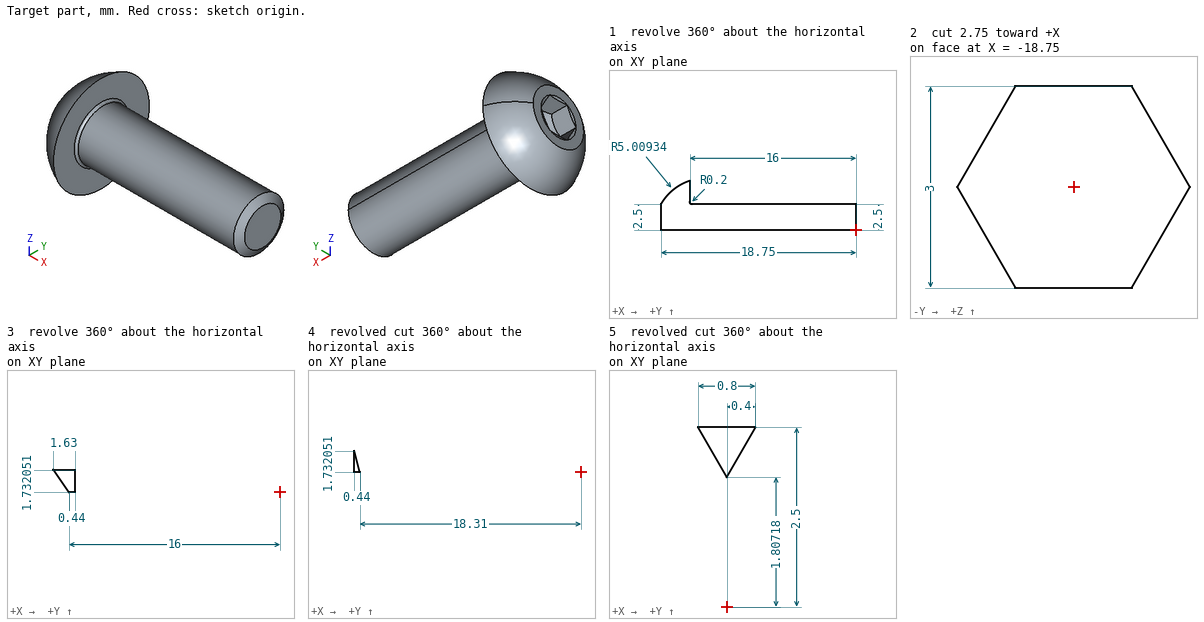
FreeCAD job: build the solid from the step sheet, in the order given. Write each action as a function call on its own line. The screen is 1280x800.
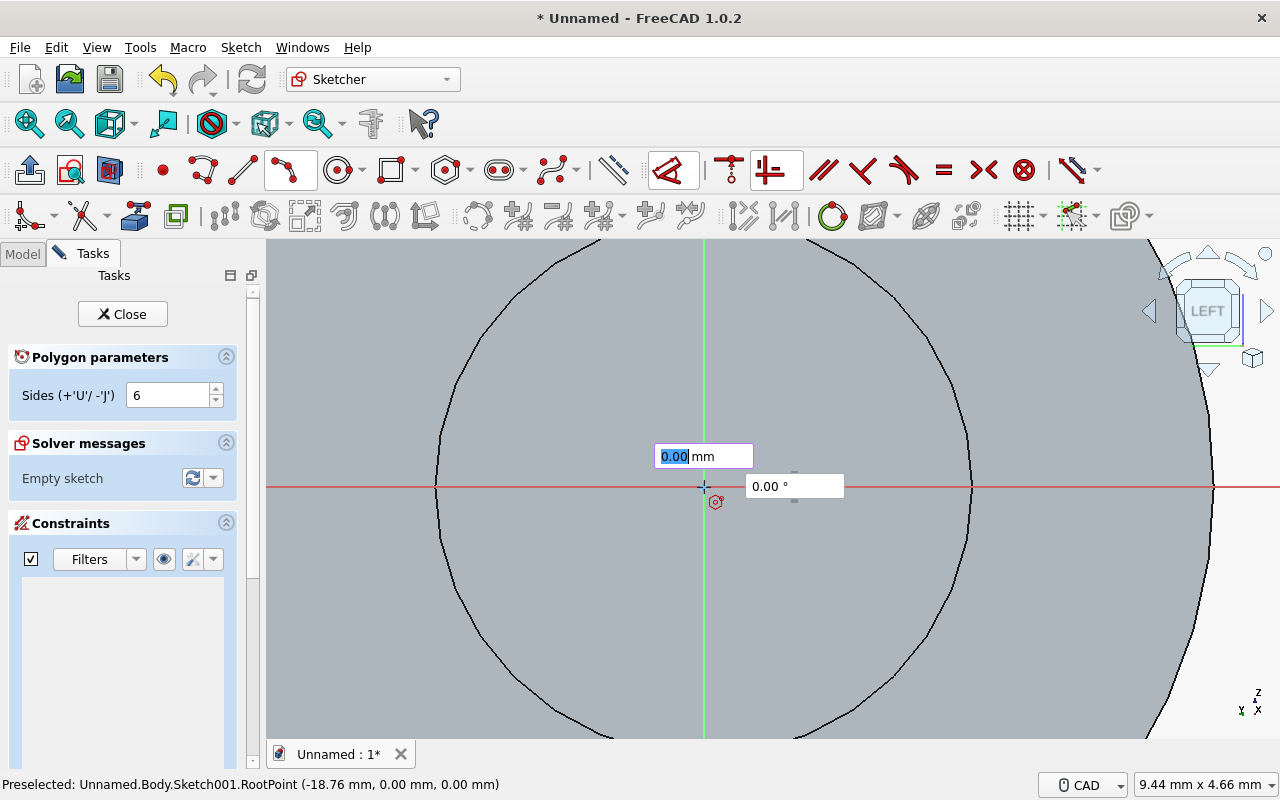
click(518, 487)
key(Escape)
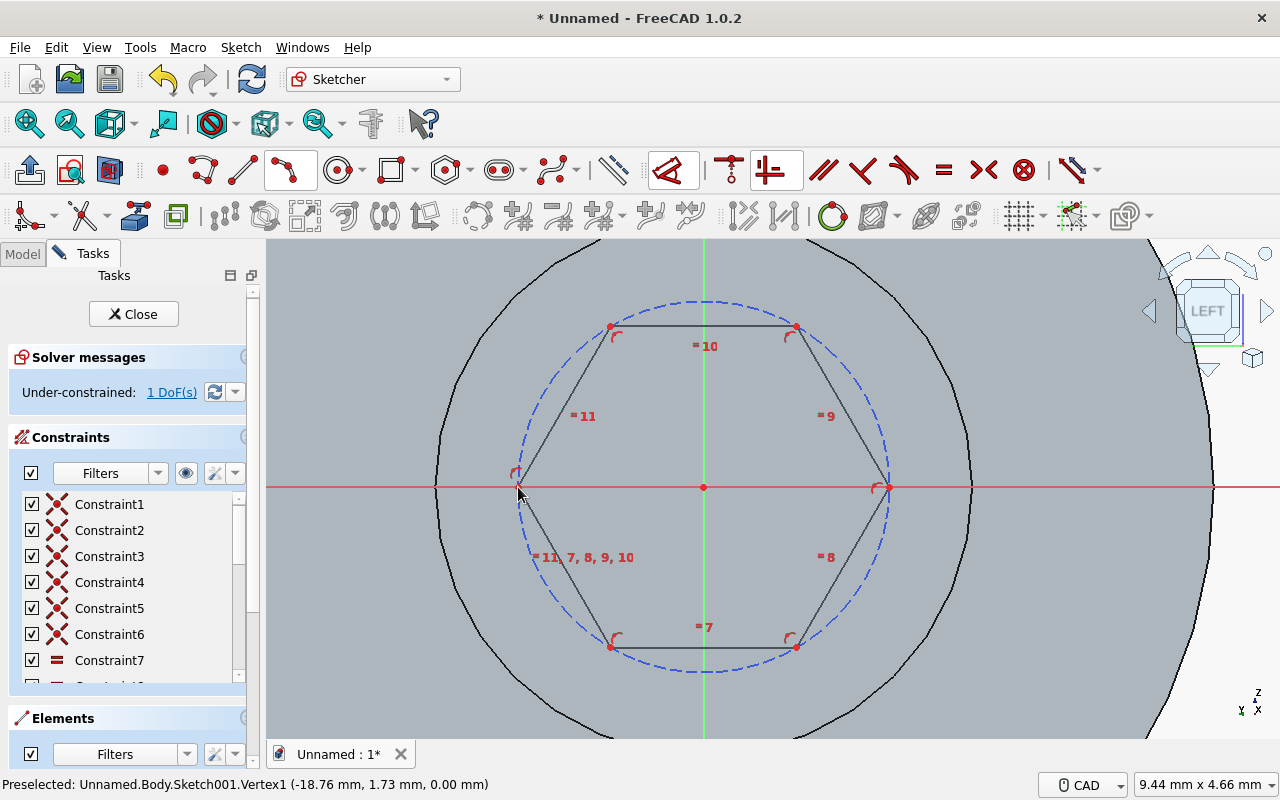
click(611, 648)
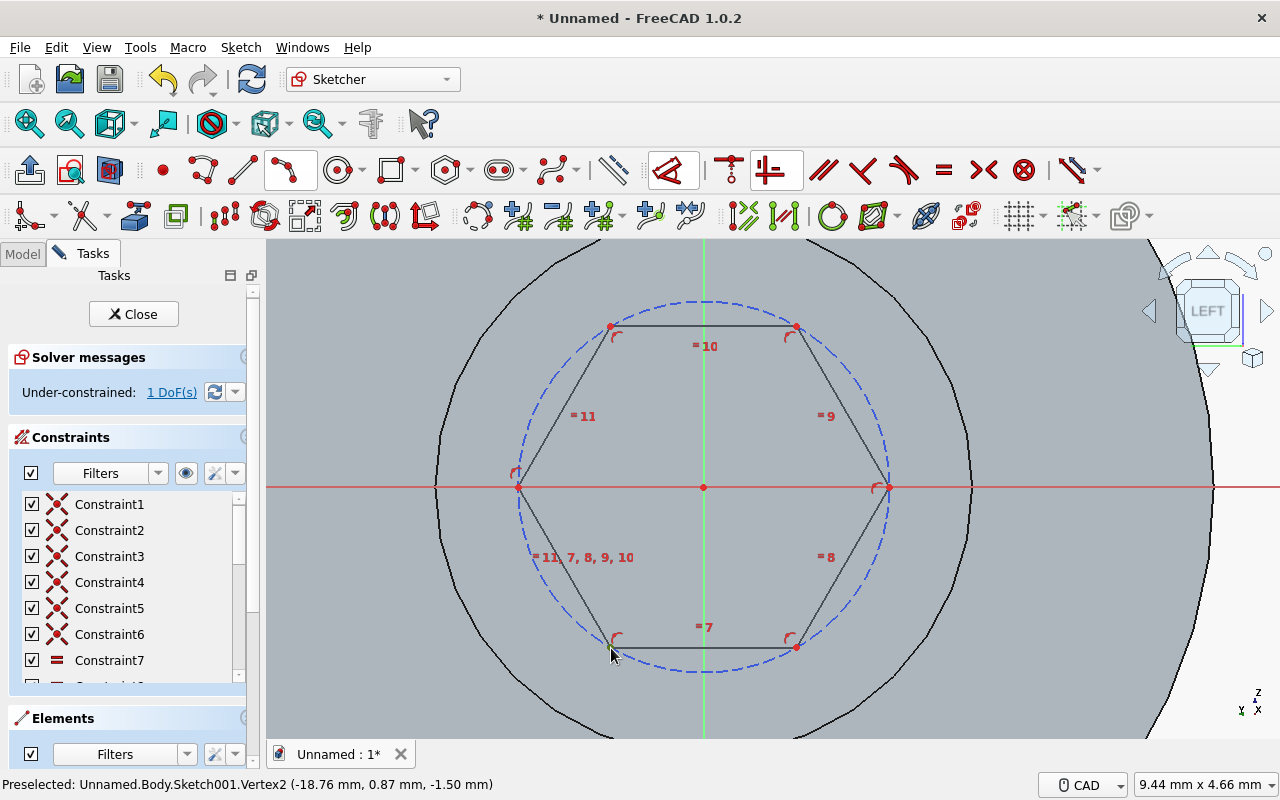
click(797, 326)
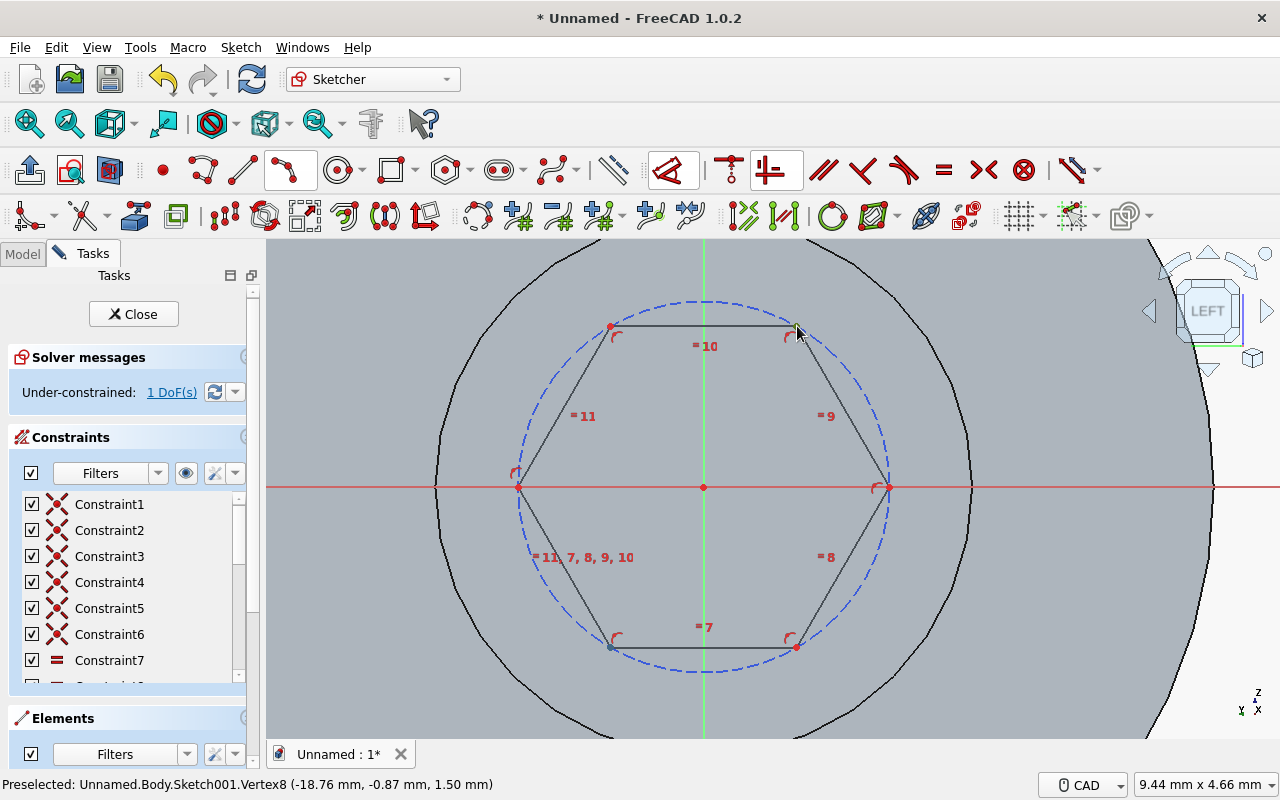
click(694, 170)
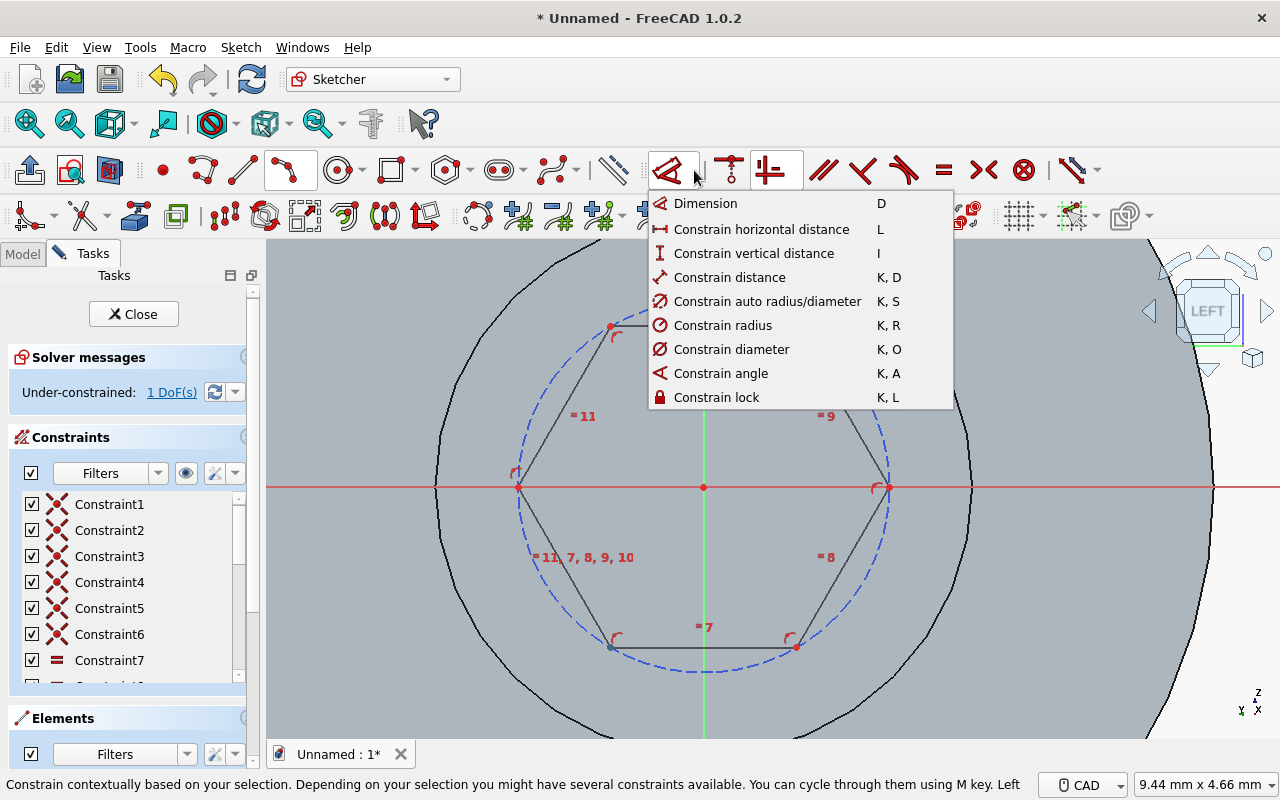
click(801, 253)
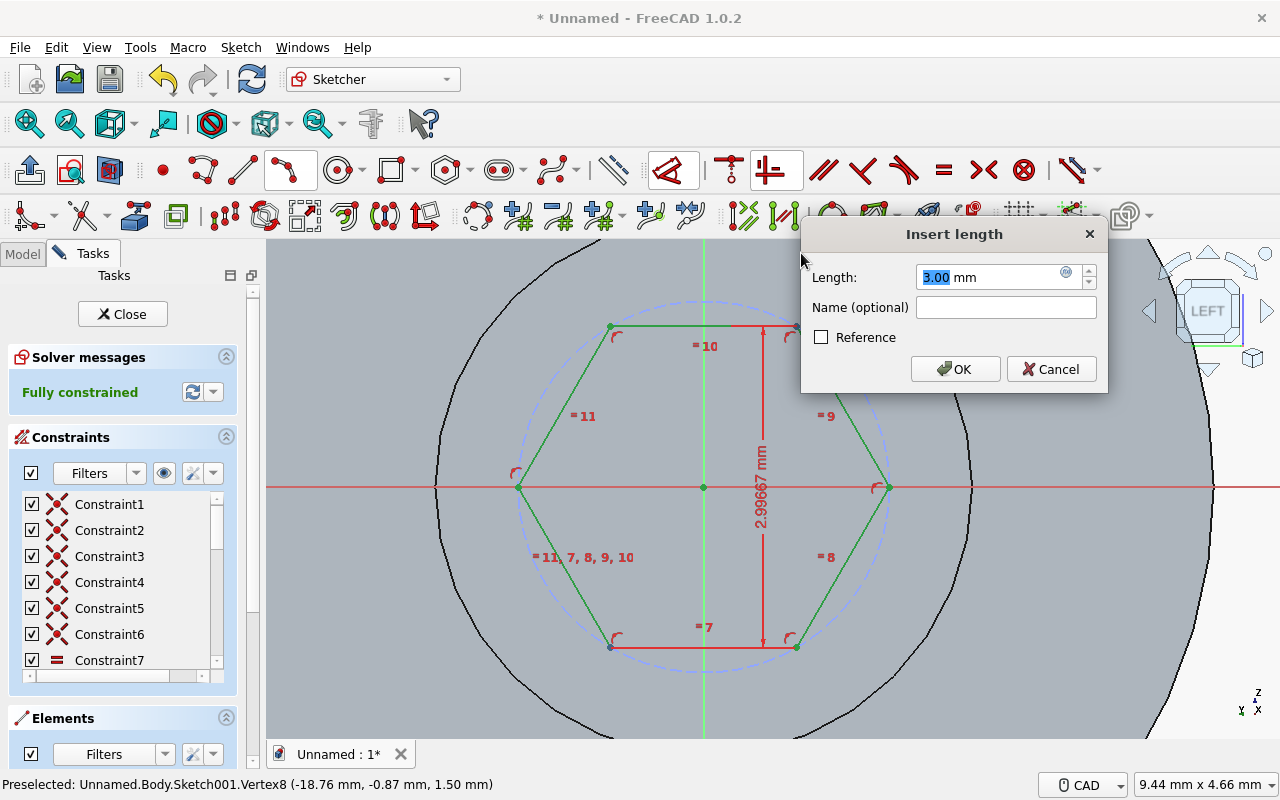
text(3)
key(Return)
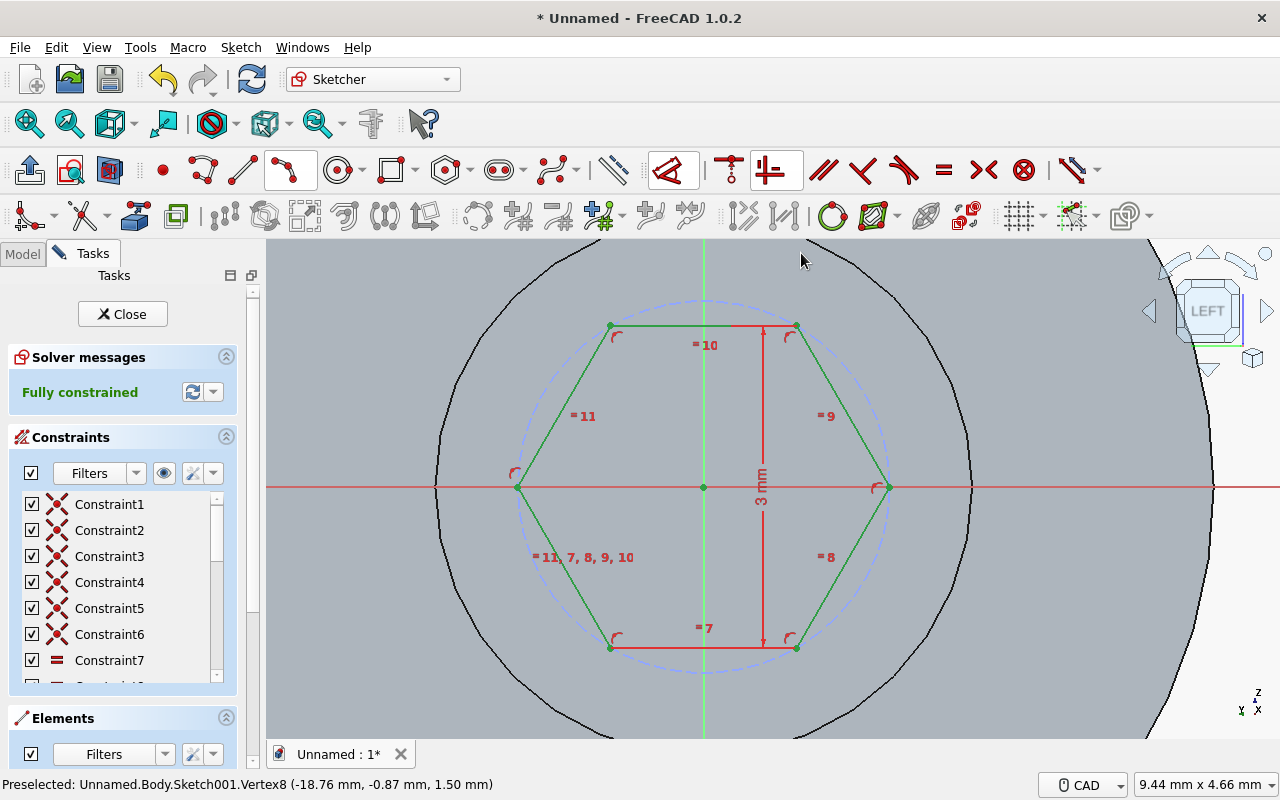
click(123, 314)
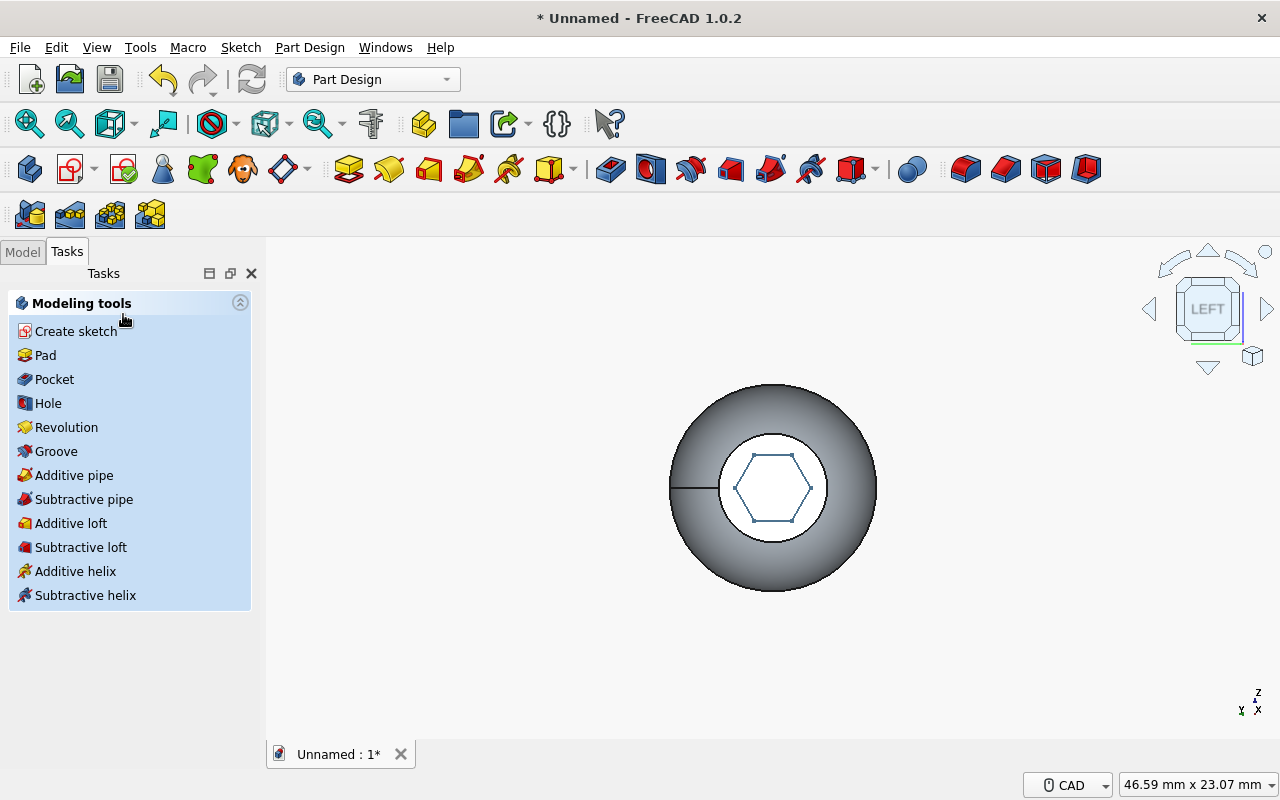
click(612, 170)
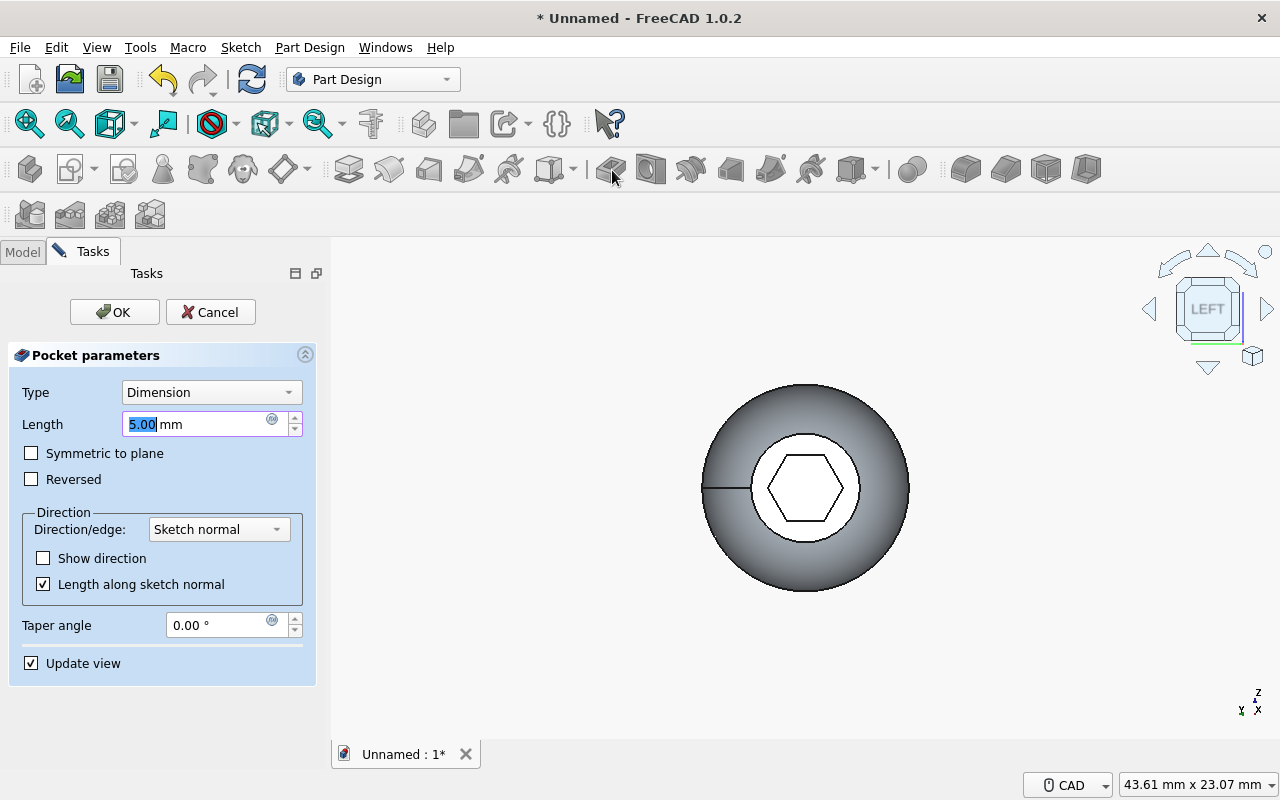
text(2.75)
key(Tab)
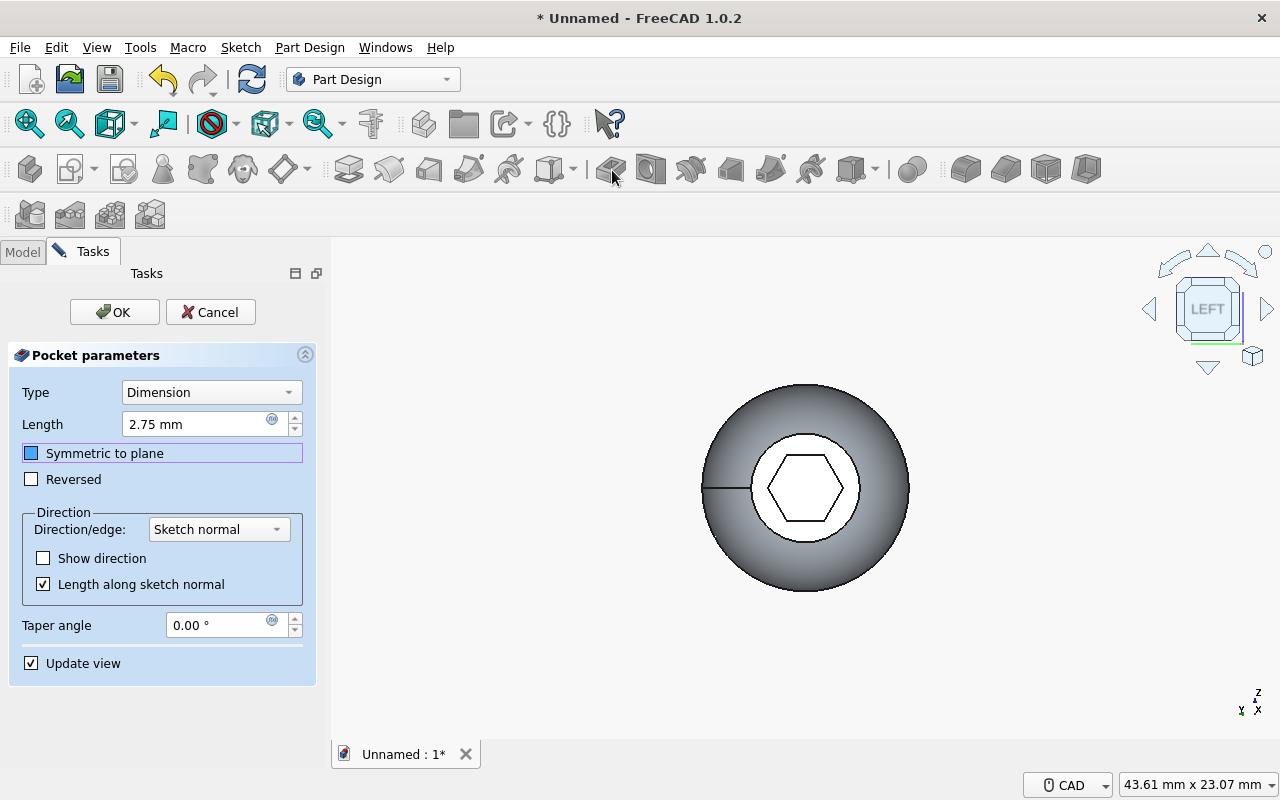
click(115, 312)